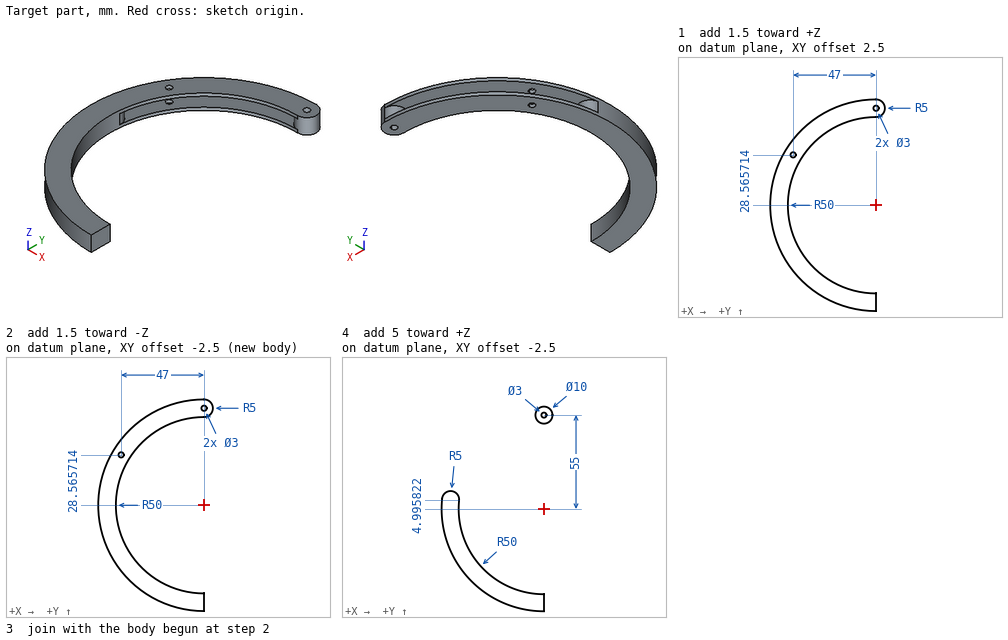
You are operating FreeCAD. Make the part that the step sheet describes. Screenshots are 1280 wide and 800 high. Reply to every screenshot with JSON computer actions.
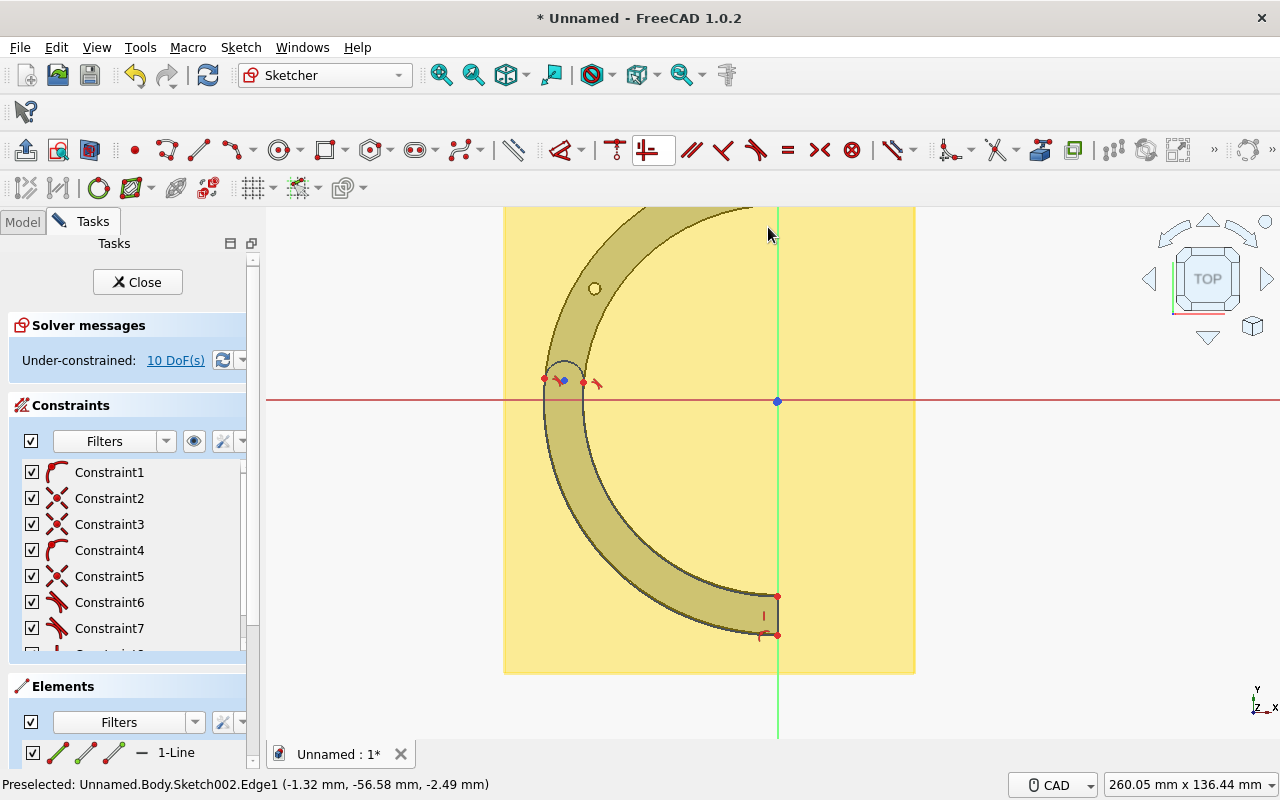
{"action": "left_click", "coordinate": [599, 478]}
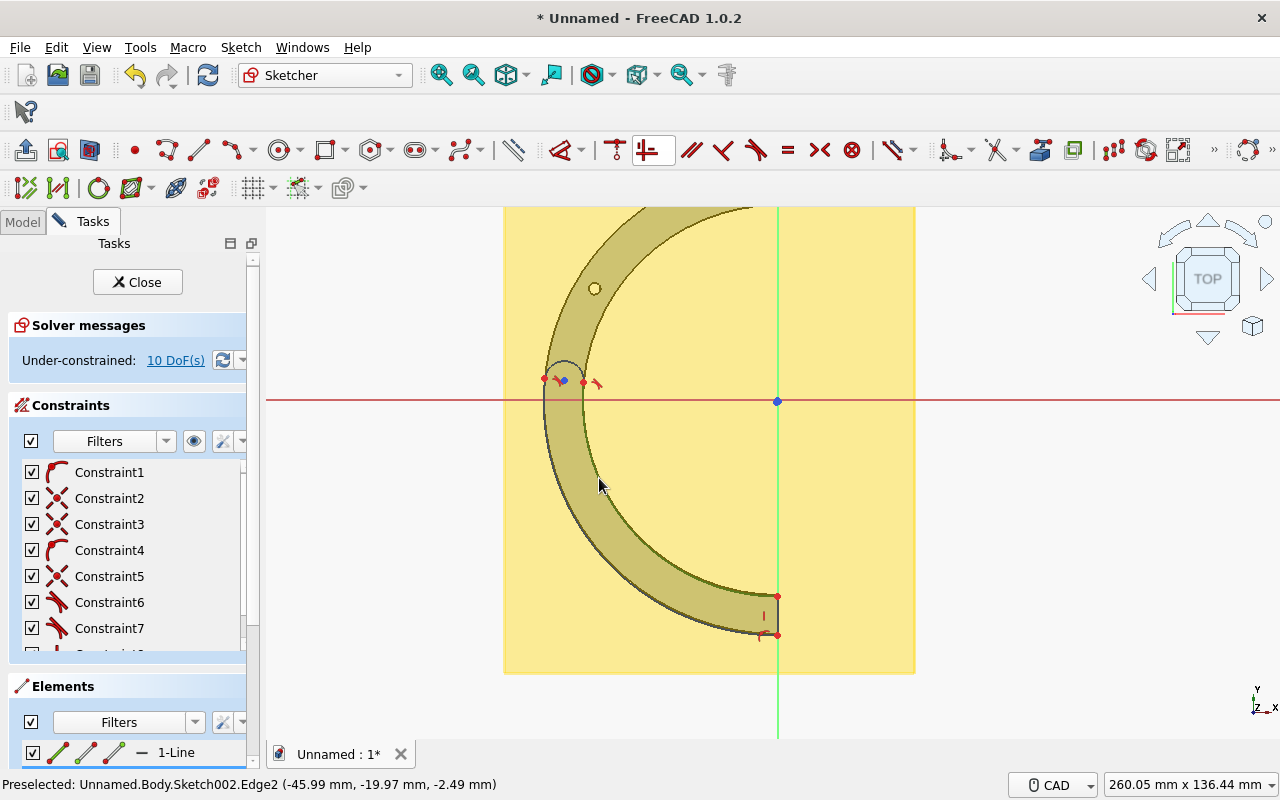
{"action": "left_click", "coordinate": [562, 493]}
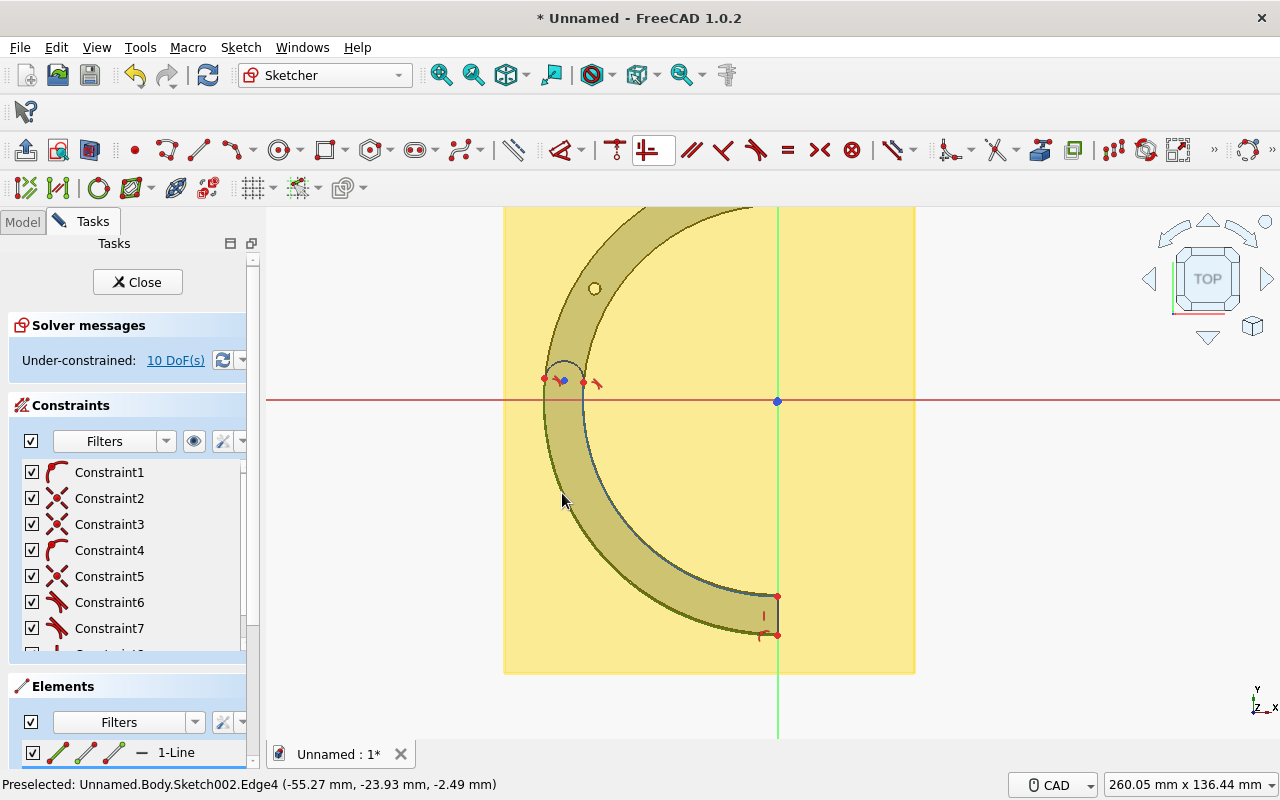
{"action": "left_click", "coordinate": [616, 150]}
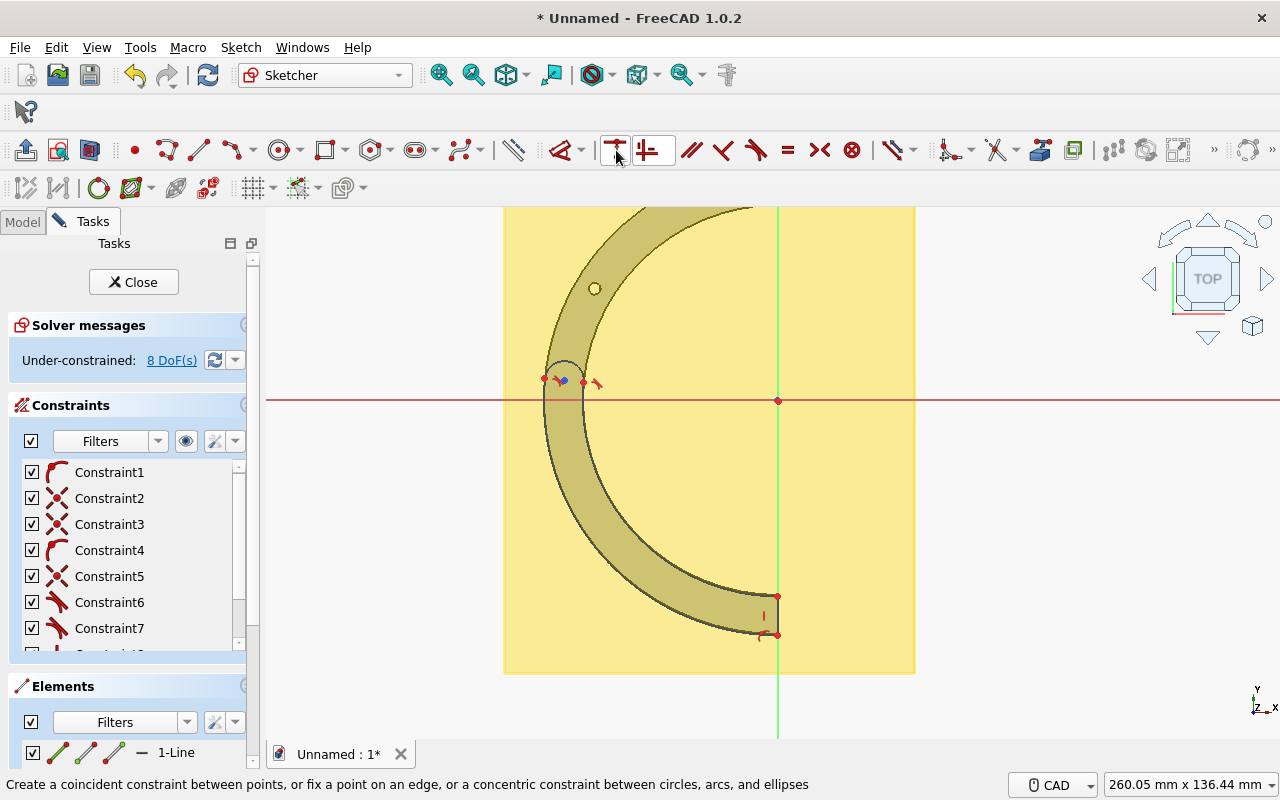
{"action": "scroll", "coordinate": [778, 401], "scroll_direction": "up", "scroll_amount": 10}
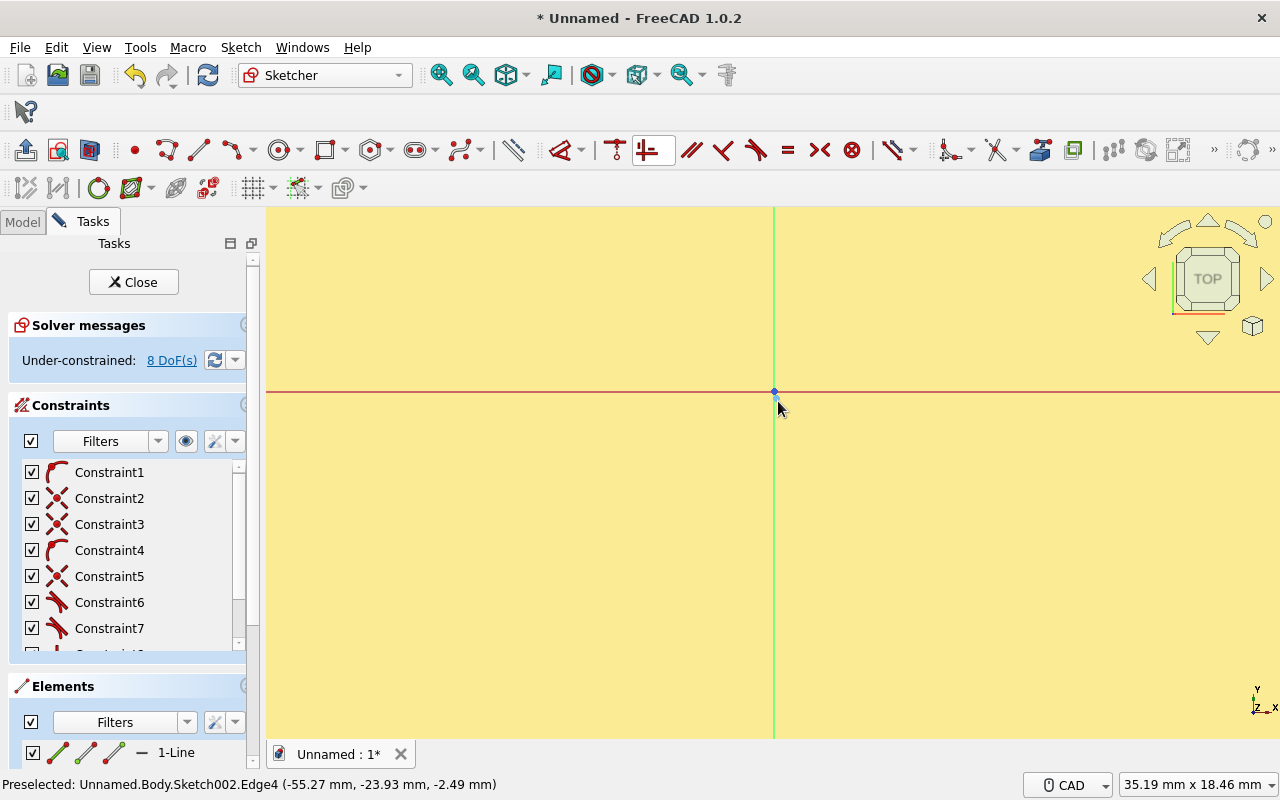
{"action": "left_click_drag", "start_coordinate": [764, 382], "coordinate": [787, 409]}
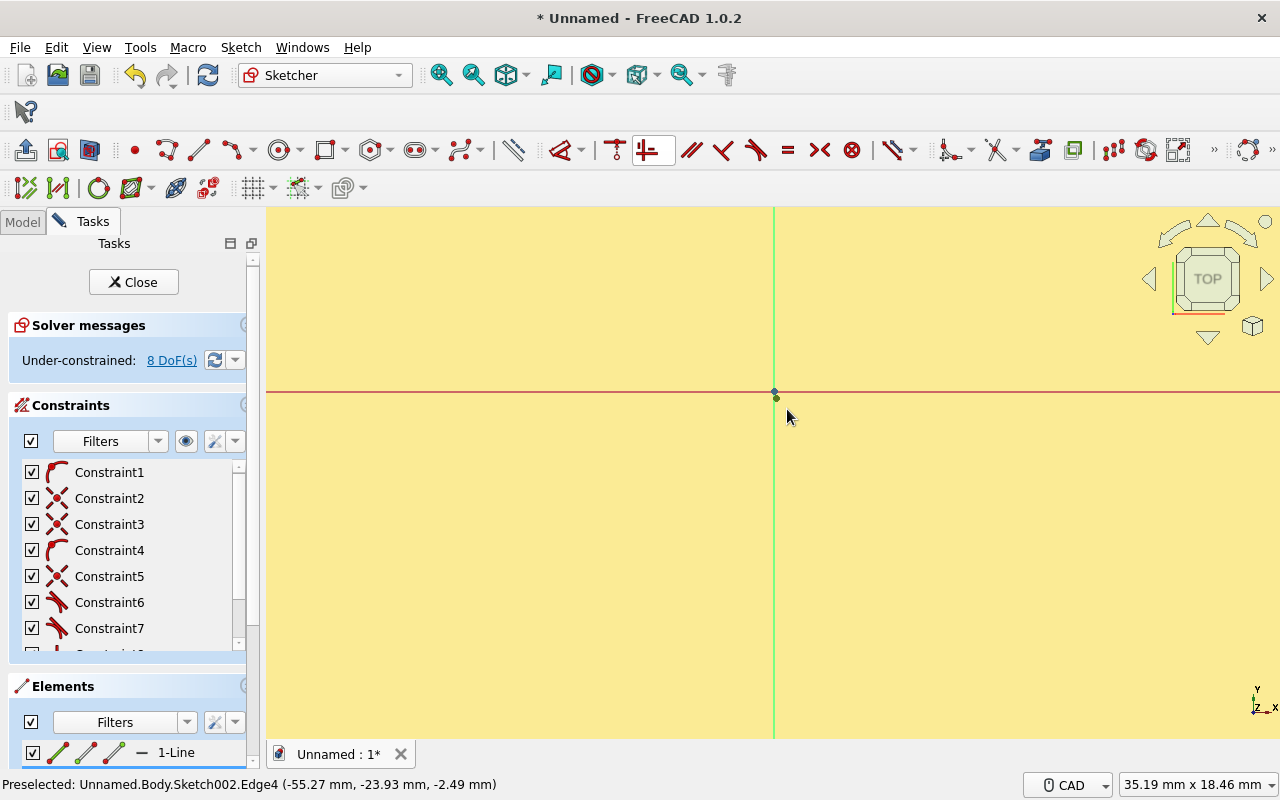
{"action": "left_click", "coordinate": [616, 150]}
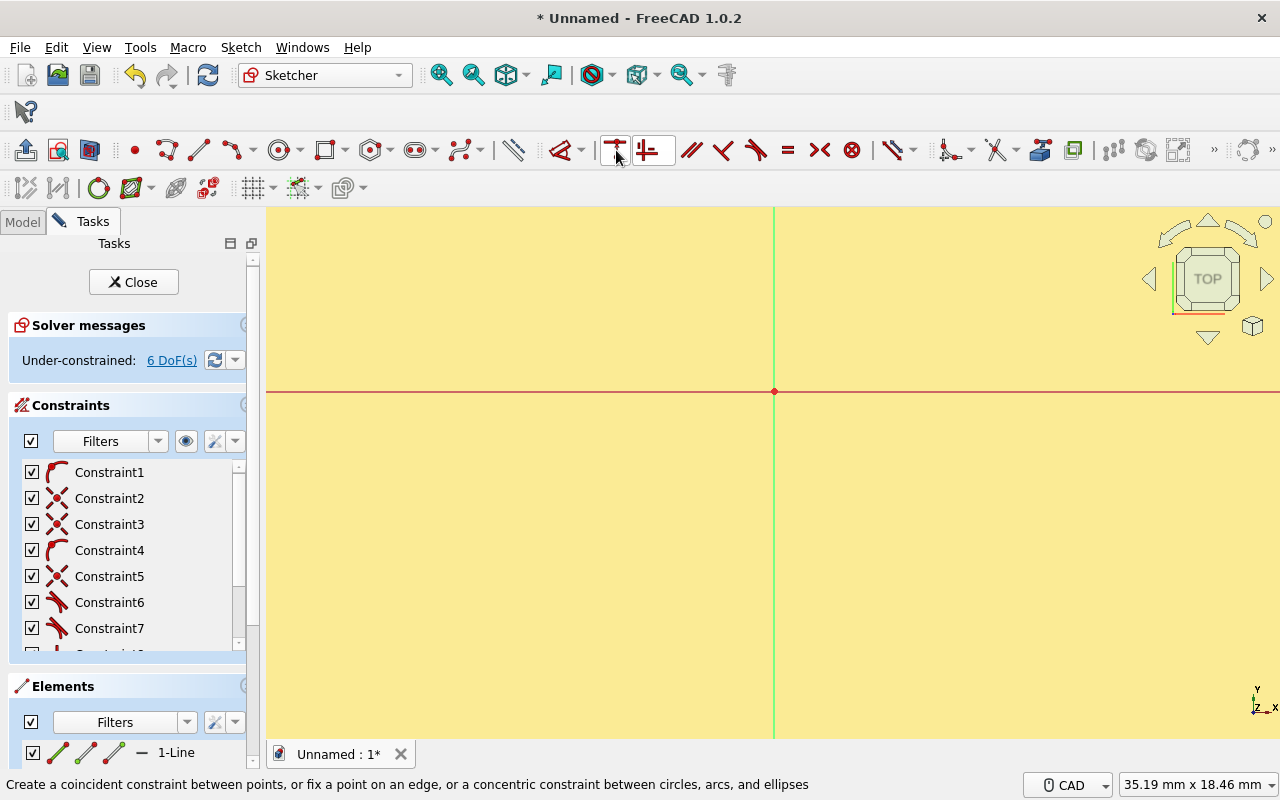
{"action": "left_click", "coordinate": [560, 150]}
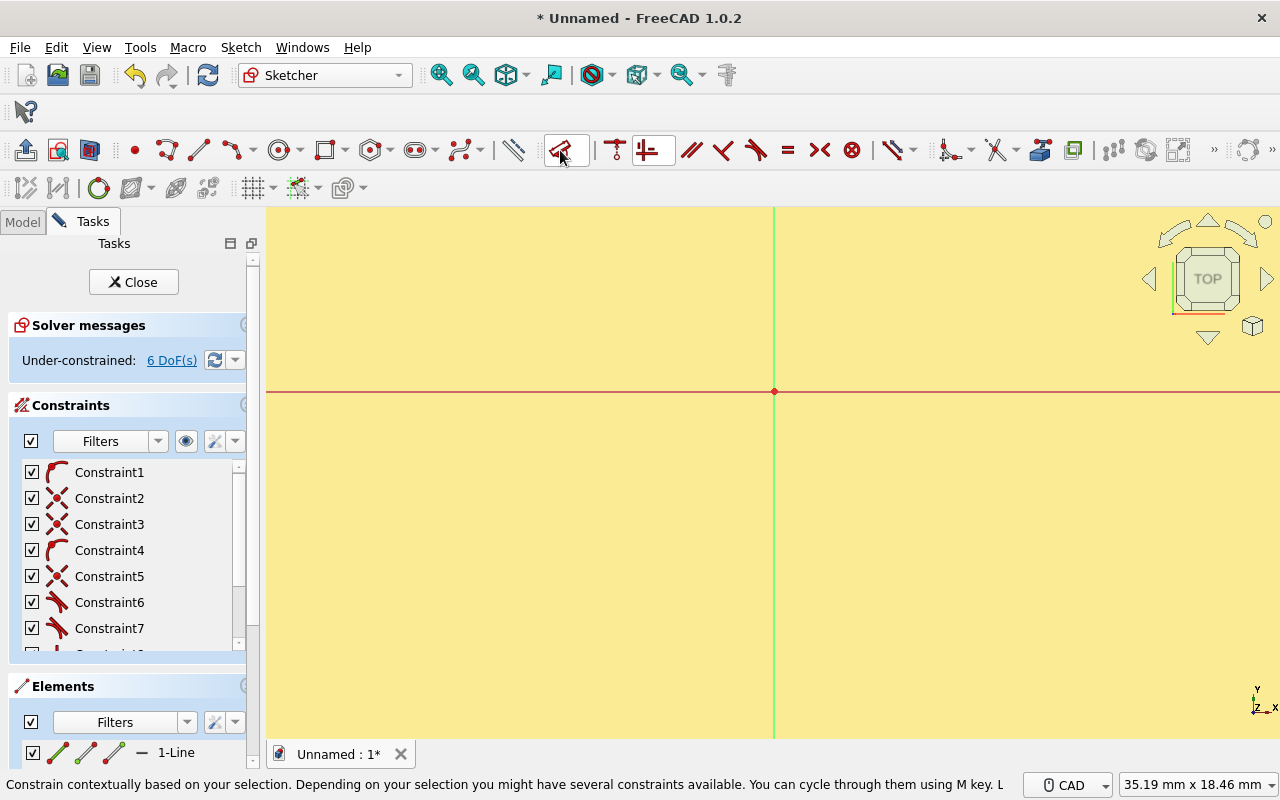
{"action": "scroll", "coordinate": [776, 481], "scroll_direction": "down", "scroll_amount": 12}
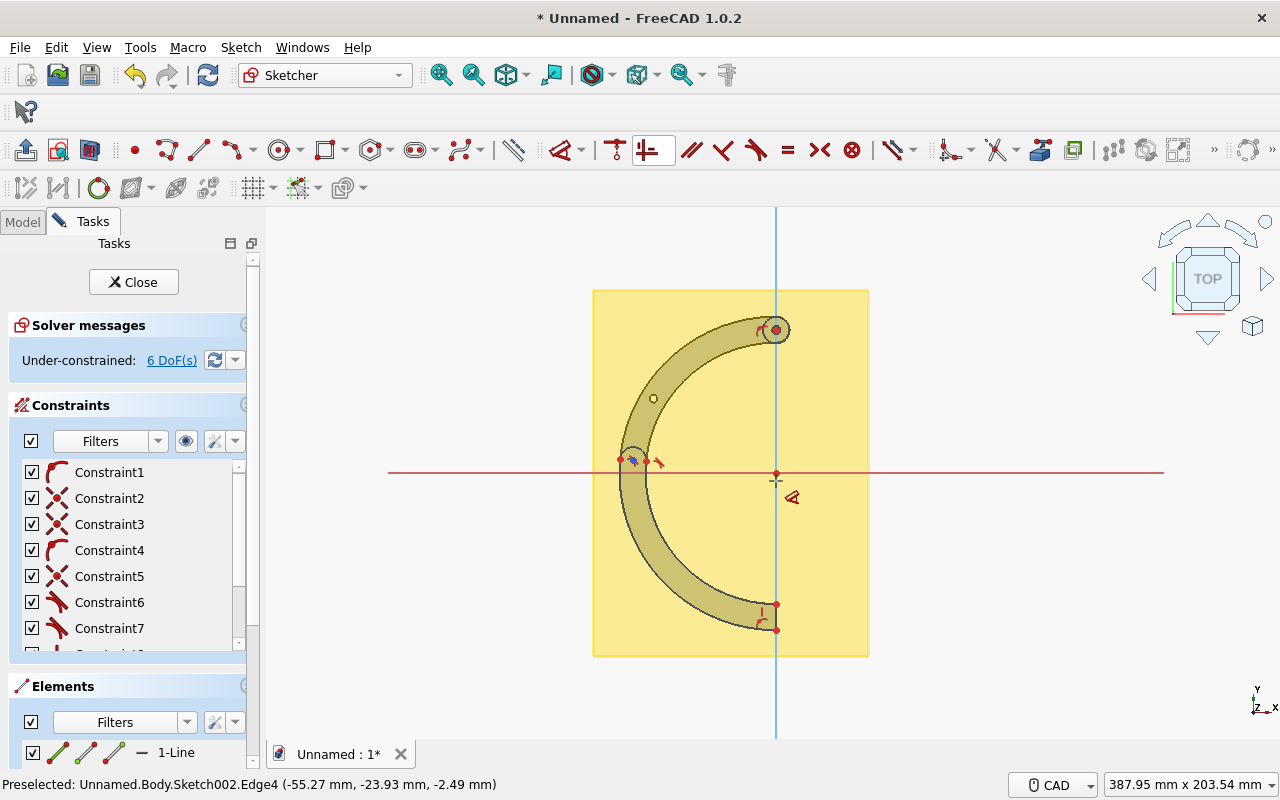
{"action": "left_click", "coordinate": [656, 525]}
{"action": "left_click", "coordinate": [641, 382]}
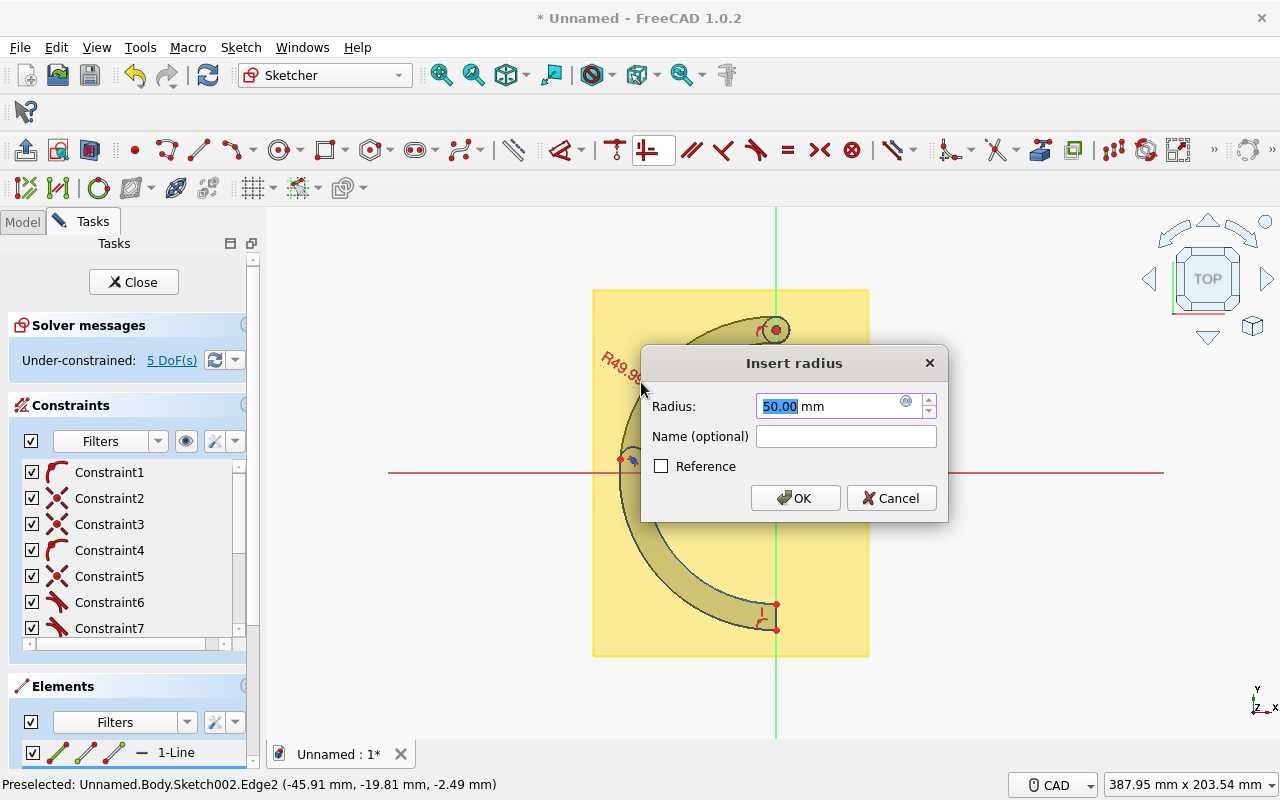
{"action": "type", "text": "50"}
{"action": "key", "text": "Return"}